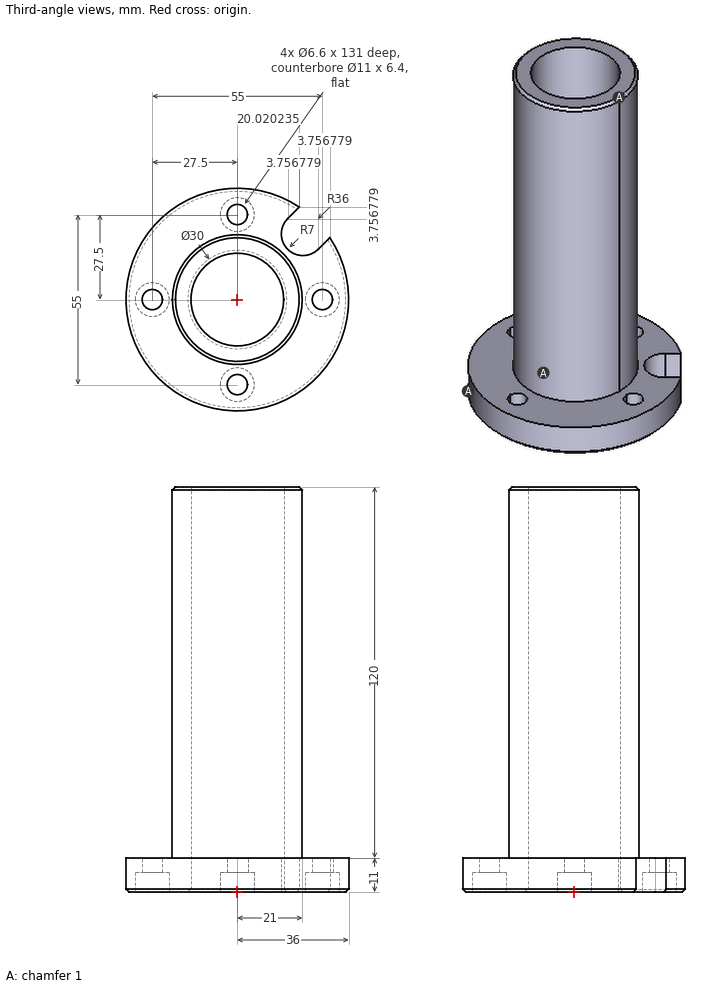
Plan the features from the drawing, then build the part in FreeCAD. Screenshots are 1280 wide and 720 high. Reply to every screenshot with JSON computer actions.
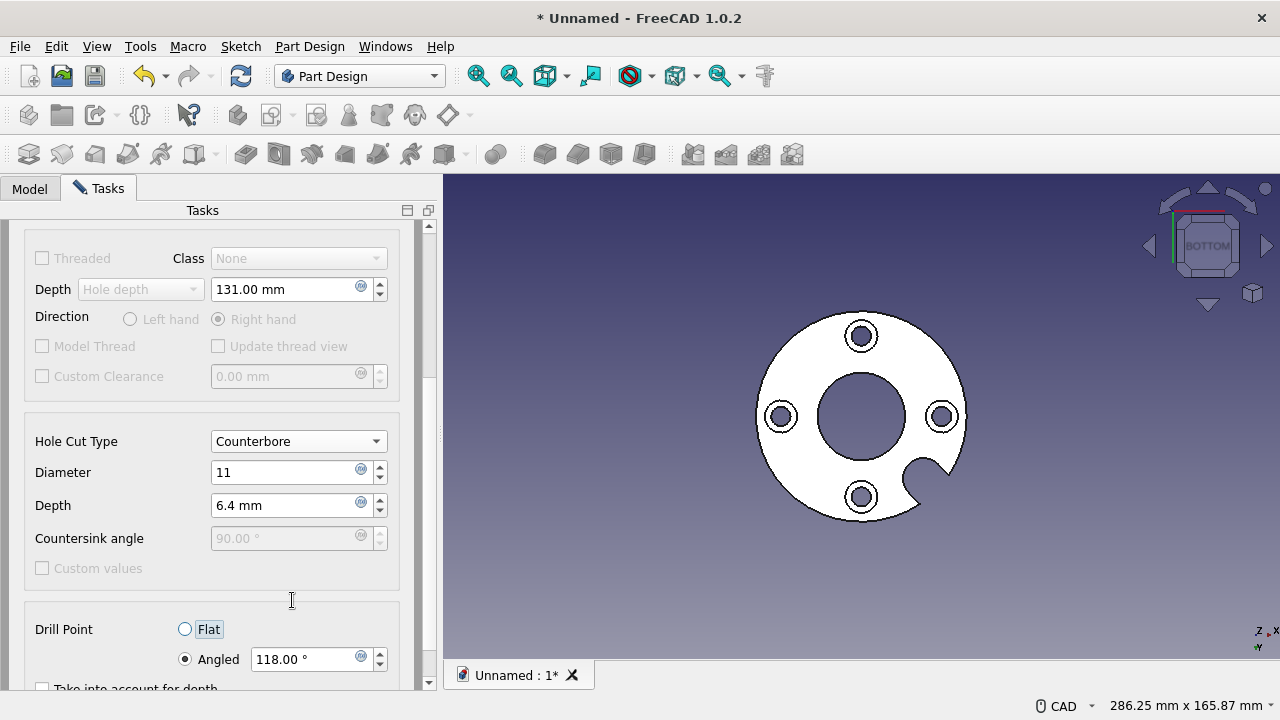
{"action": "left_click", "coordinate": [186, 627]}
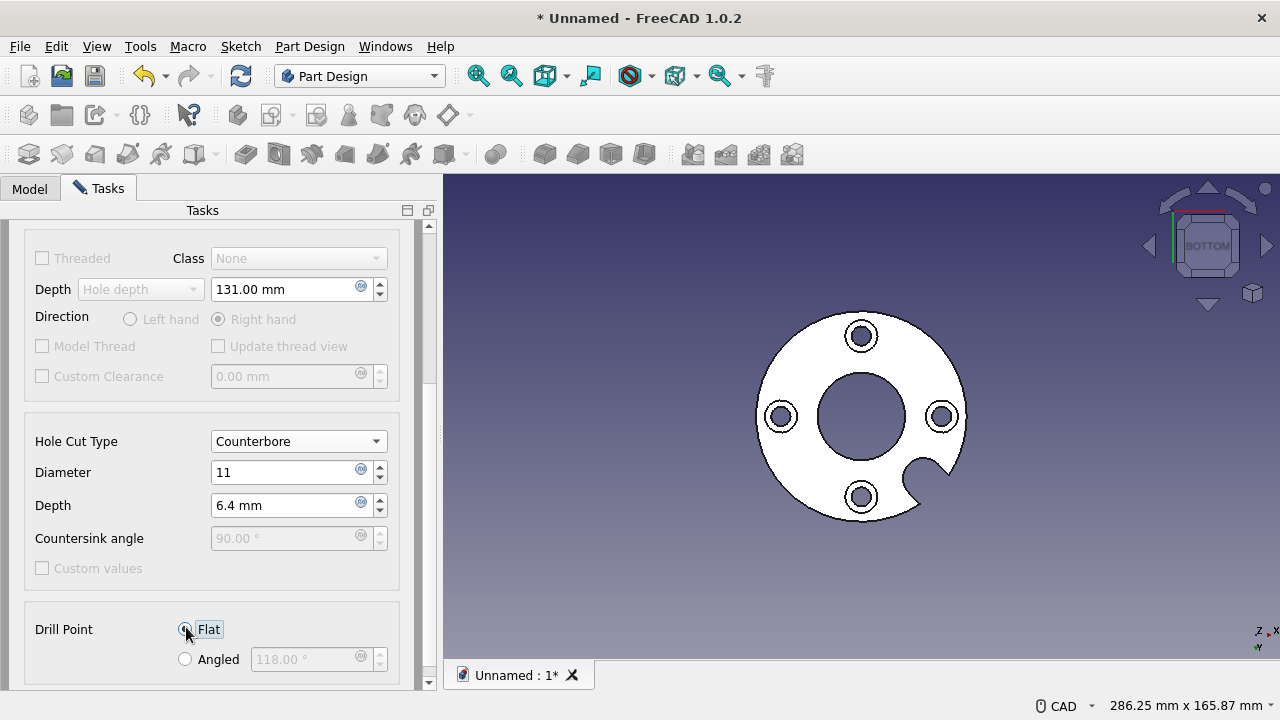
{"action": "scroll", "coordinate": [429, 455], "scroll_direction": "up", "scroll_amount": 5}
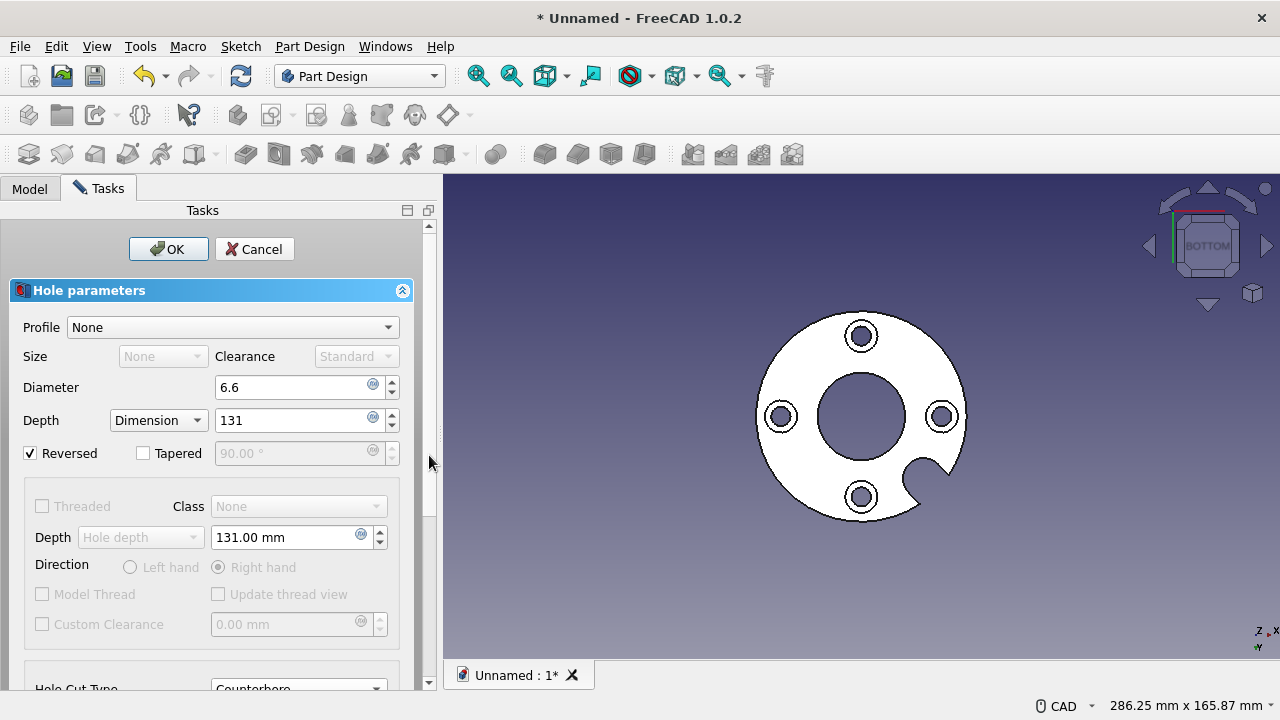
{"action": "left_click", "coordinate": [169, 249]}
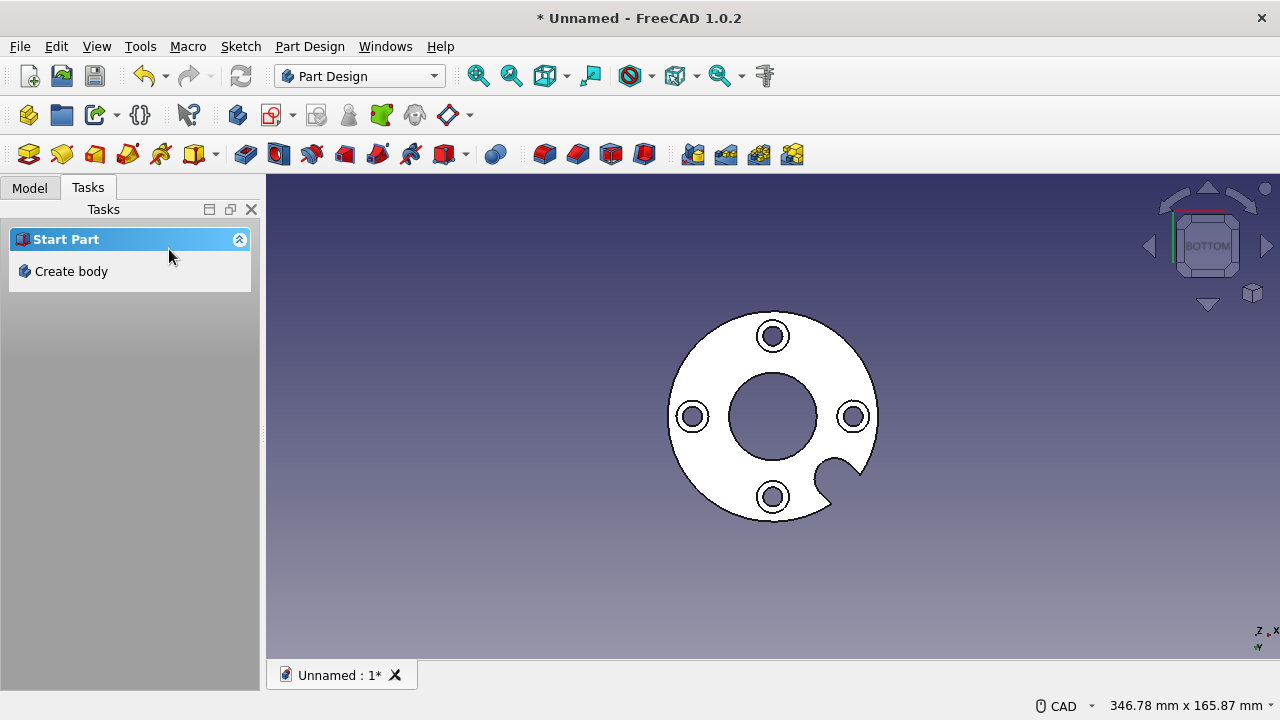
{"action": "left_click", "coordinate": [479, 76]}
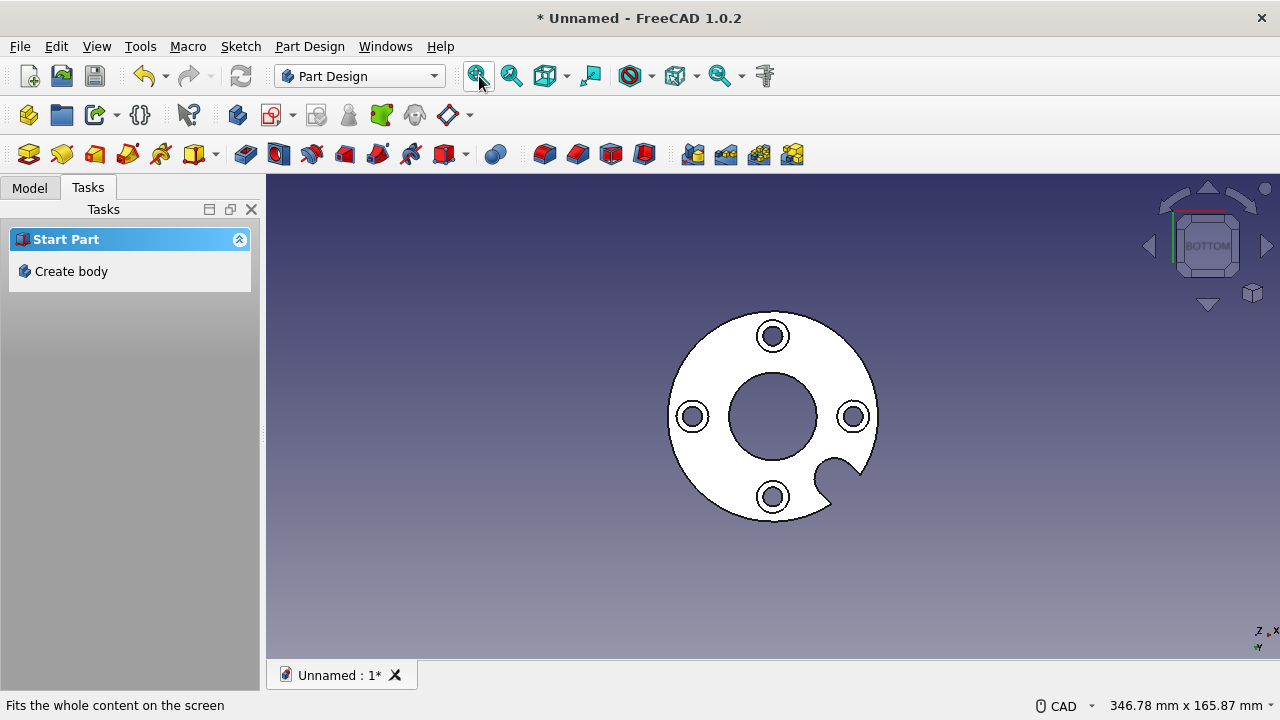
{"action": "left_click", "coordinate": [680, 366]}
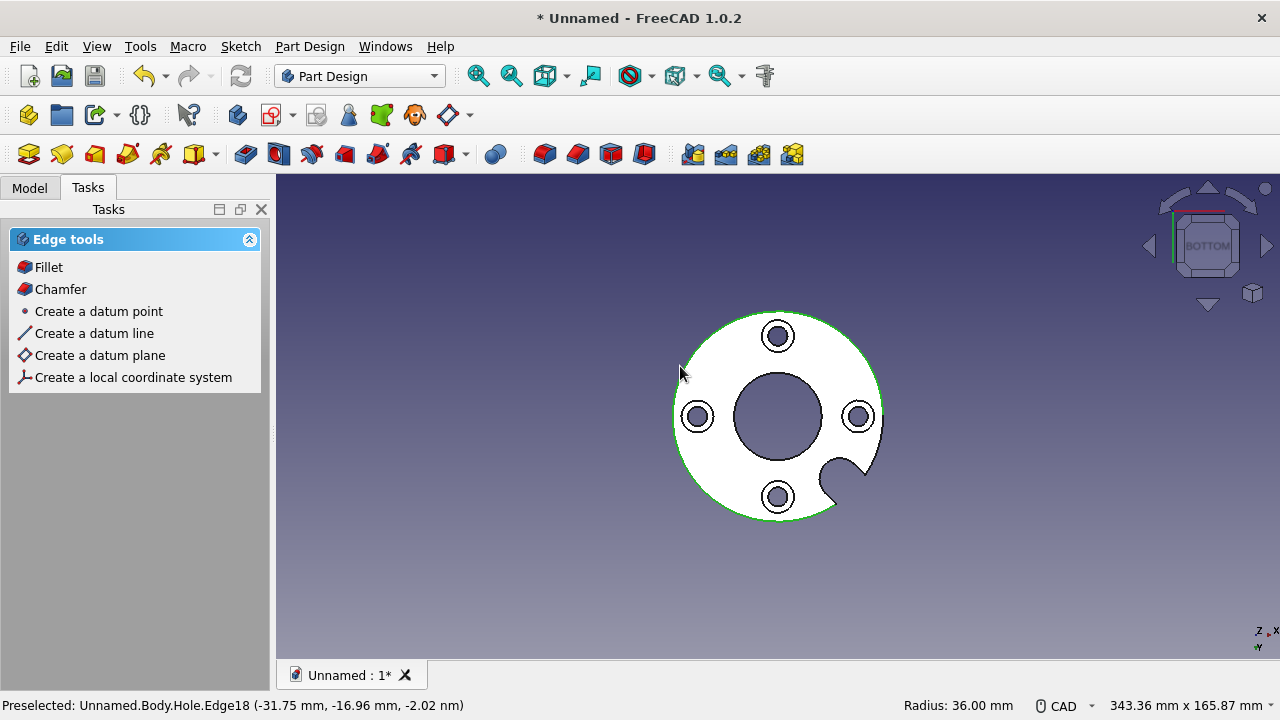
{"action": "left_click", "coordinate": [734, 415], "text": "ctrl"}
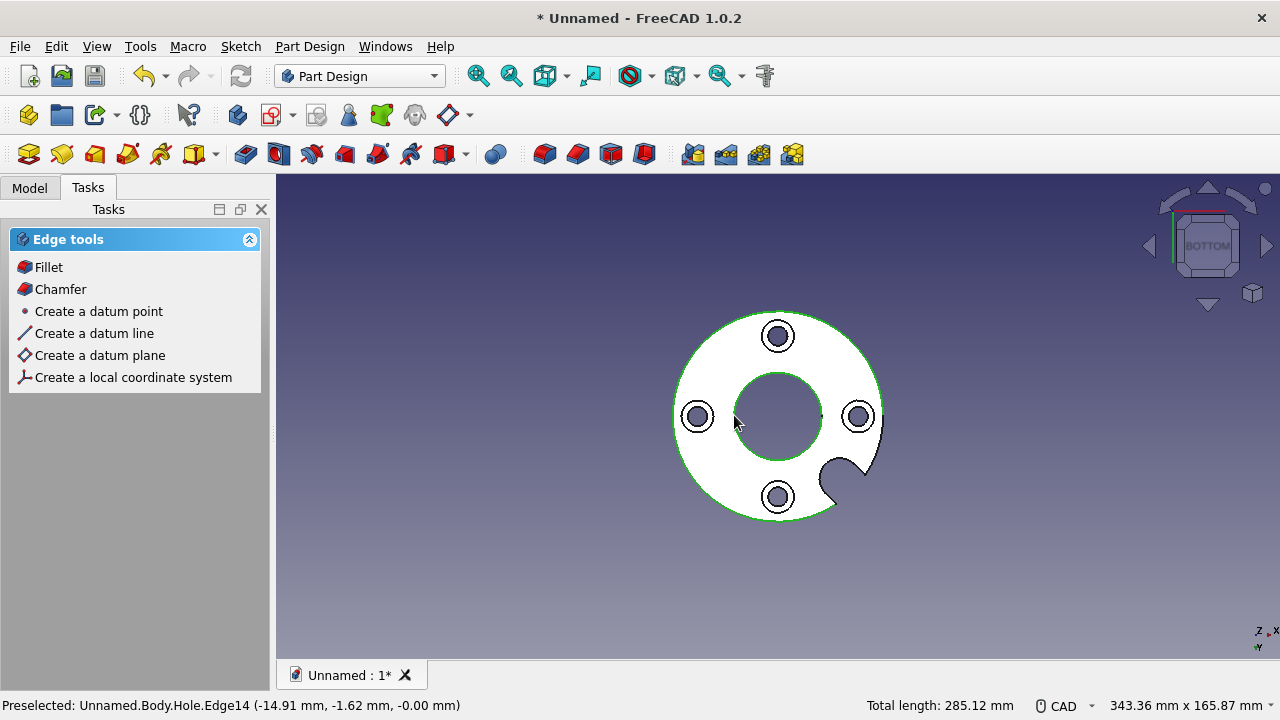
{"action": "key", "text": "0"}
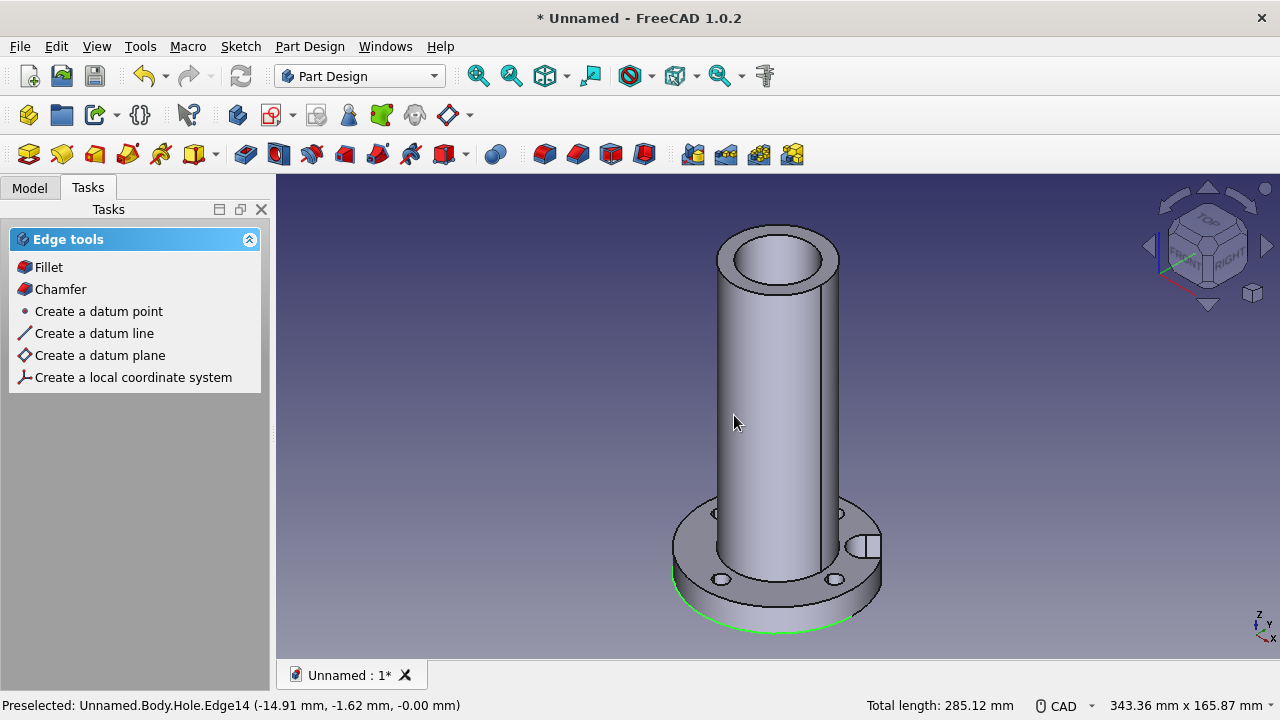
{"action": "key", "text": "v f"}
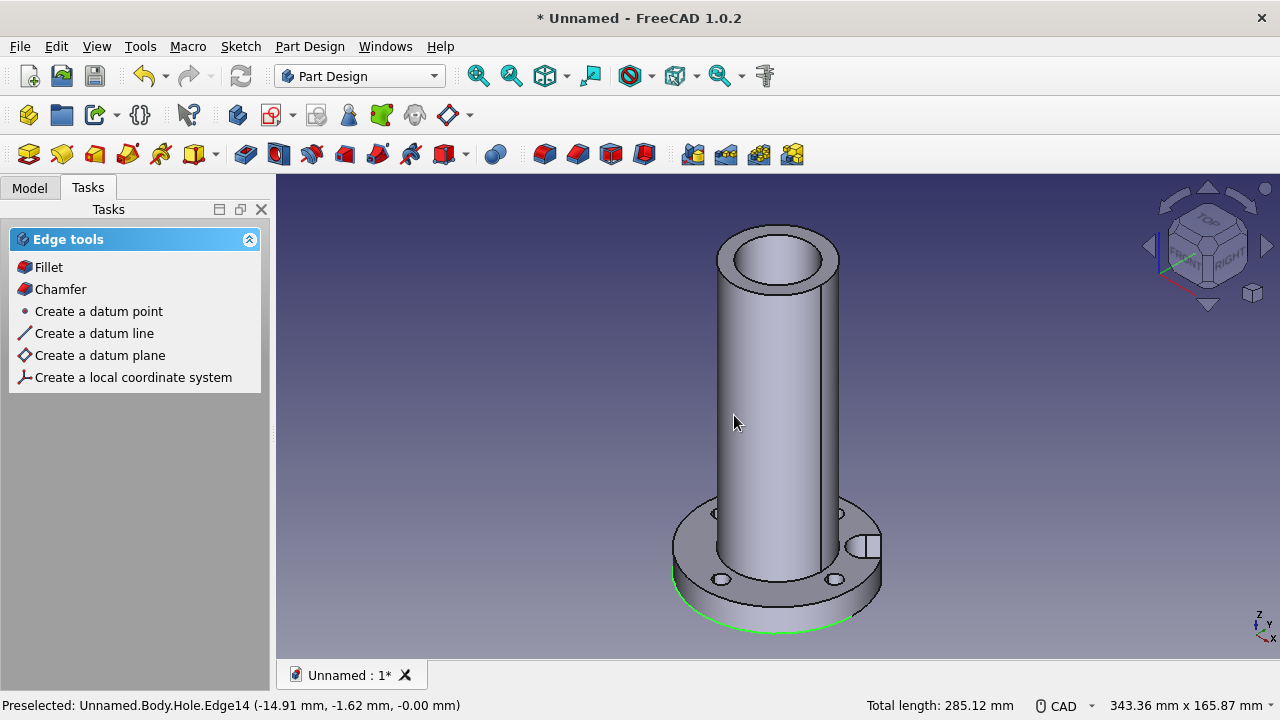
{"action": "left_click", "coordinate": [723, 275], "text": "ctrl"}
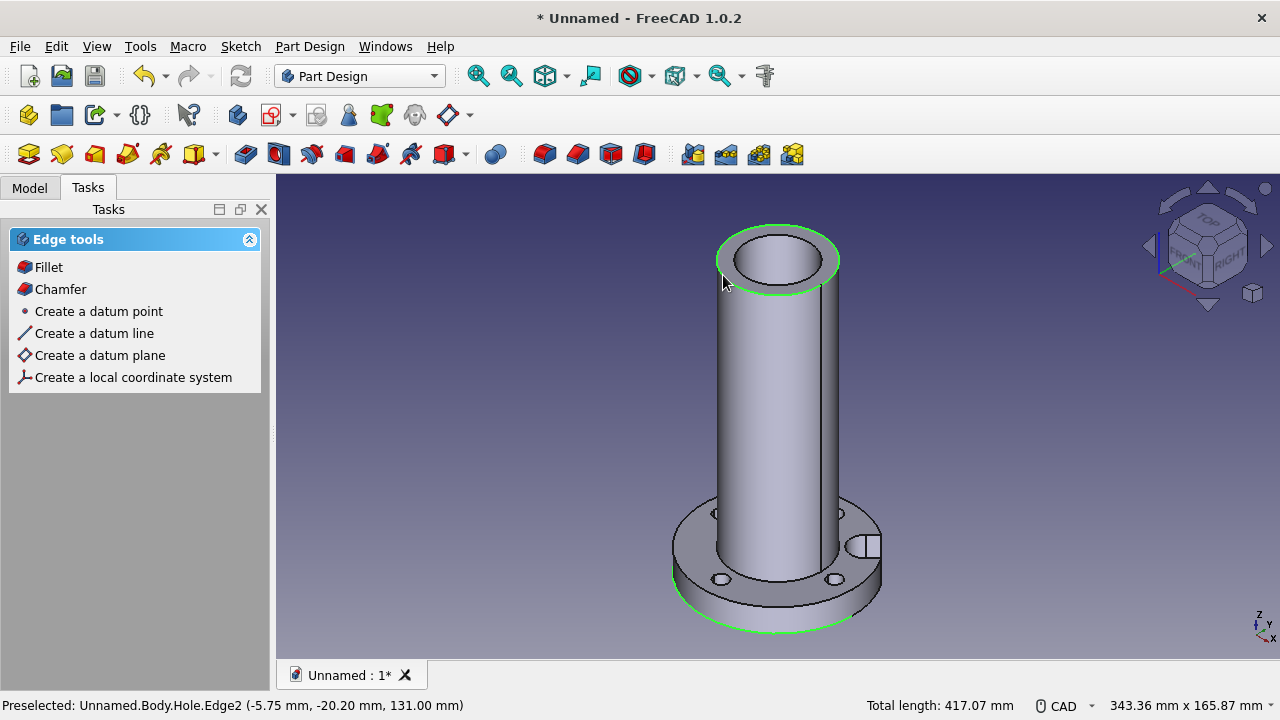
{"action": "left_click", "coordinate": [578, 154]}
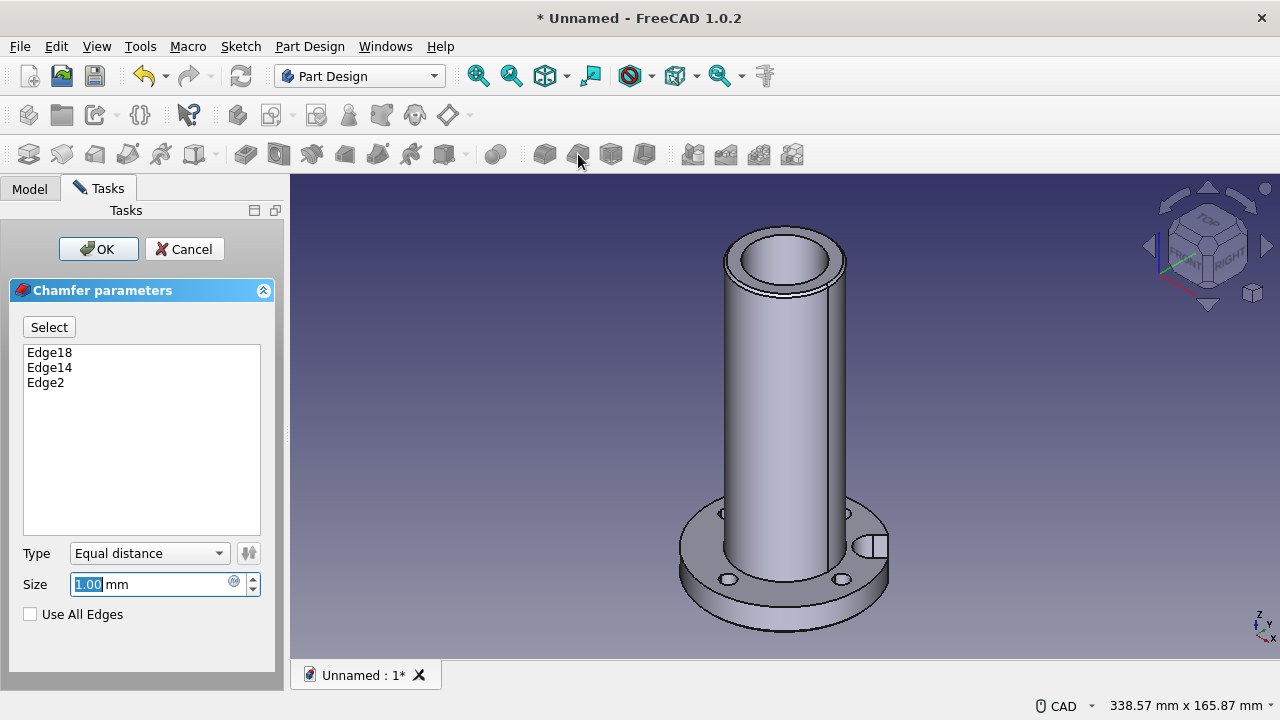
{"action": "type", "text": "1"}
{"action": "key", "text": "Tab"}